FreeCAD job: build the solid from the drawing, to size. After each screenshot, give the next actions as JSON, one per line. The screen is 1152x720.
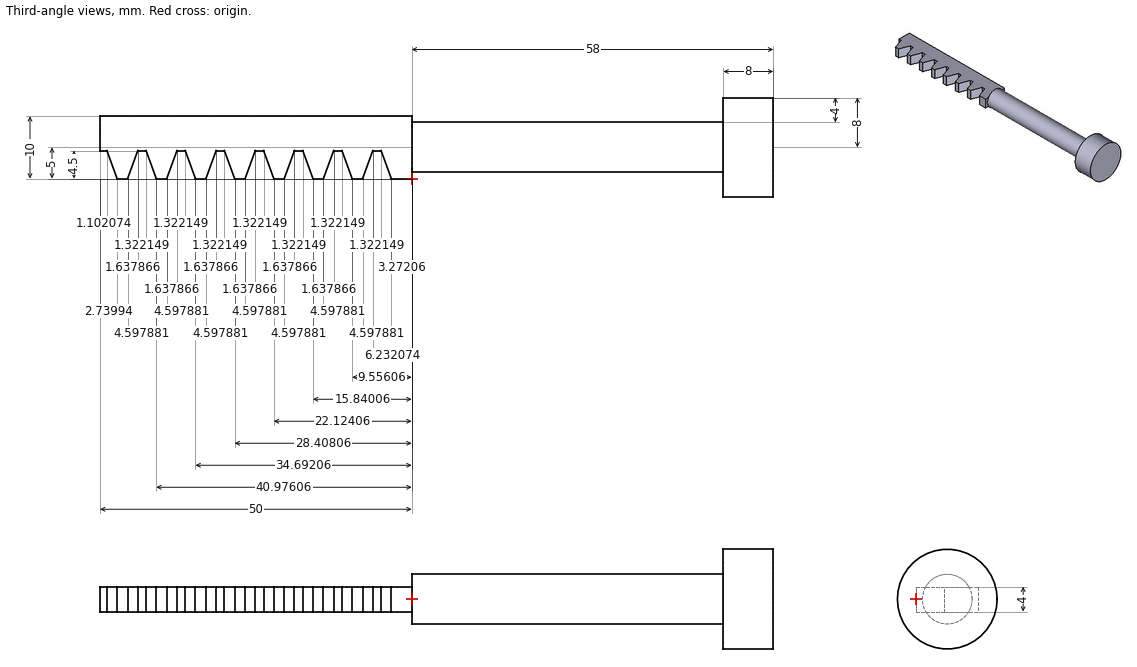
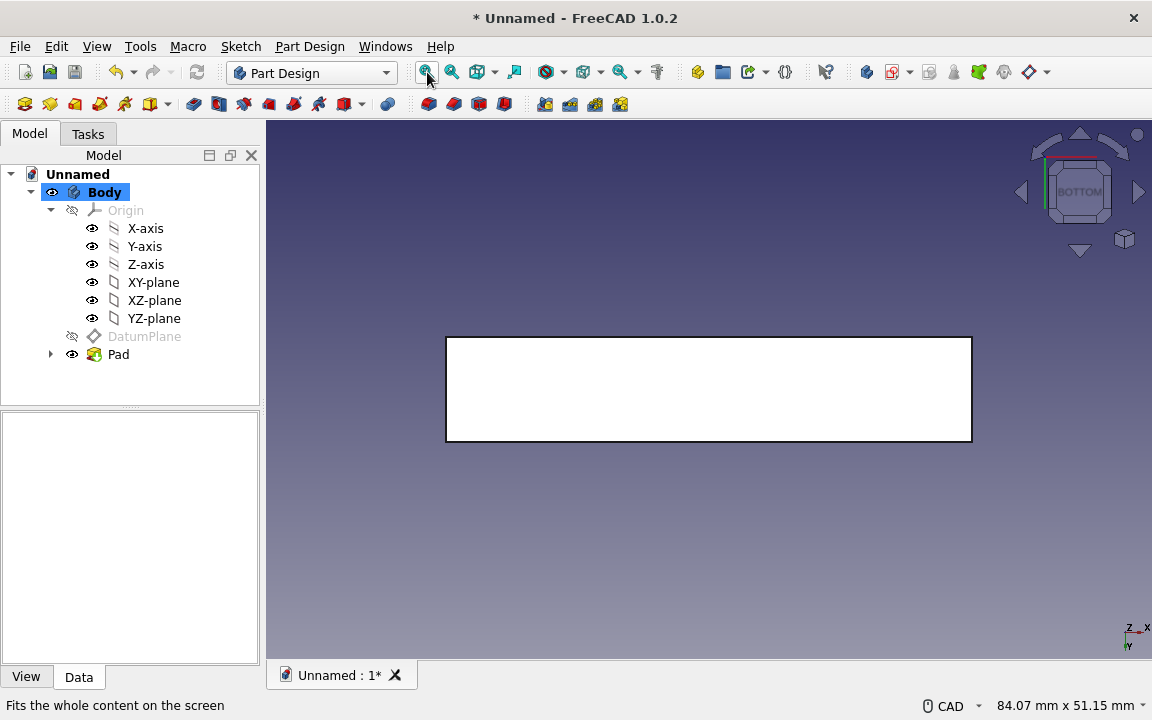
{"action": "left_click", "coordinate": [860, 388]}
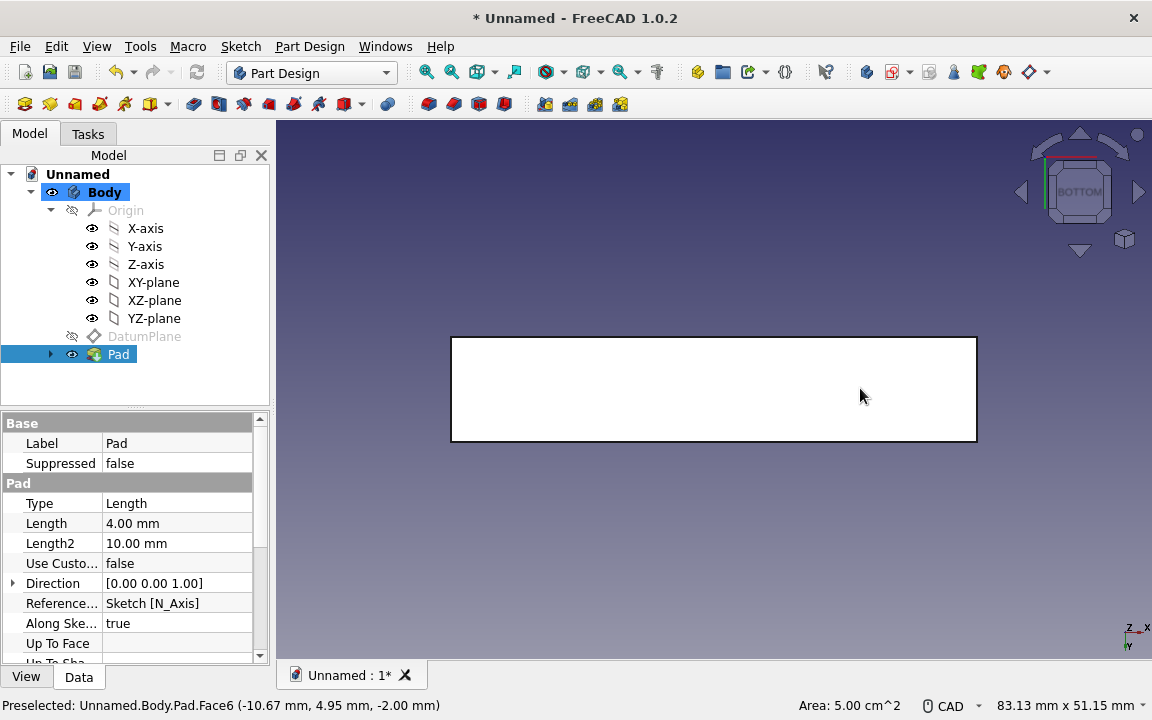
{"action": "left_click", "coordinate": [892, 72]}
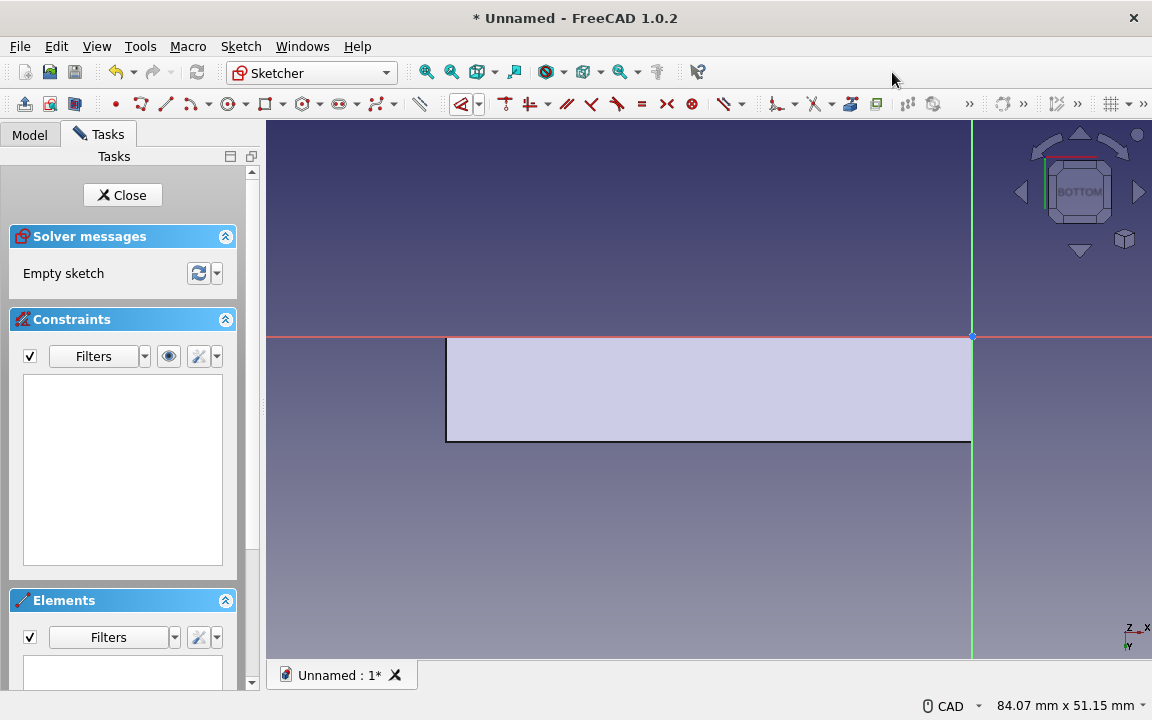
{"action": "scroll", "coordinate": [497, 356], "scroll_direction": "up", "scroll_amount": 10}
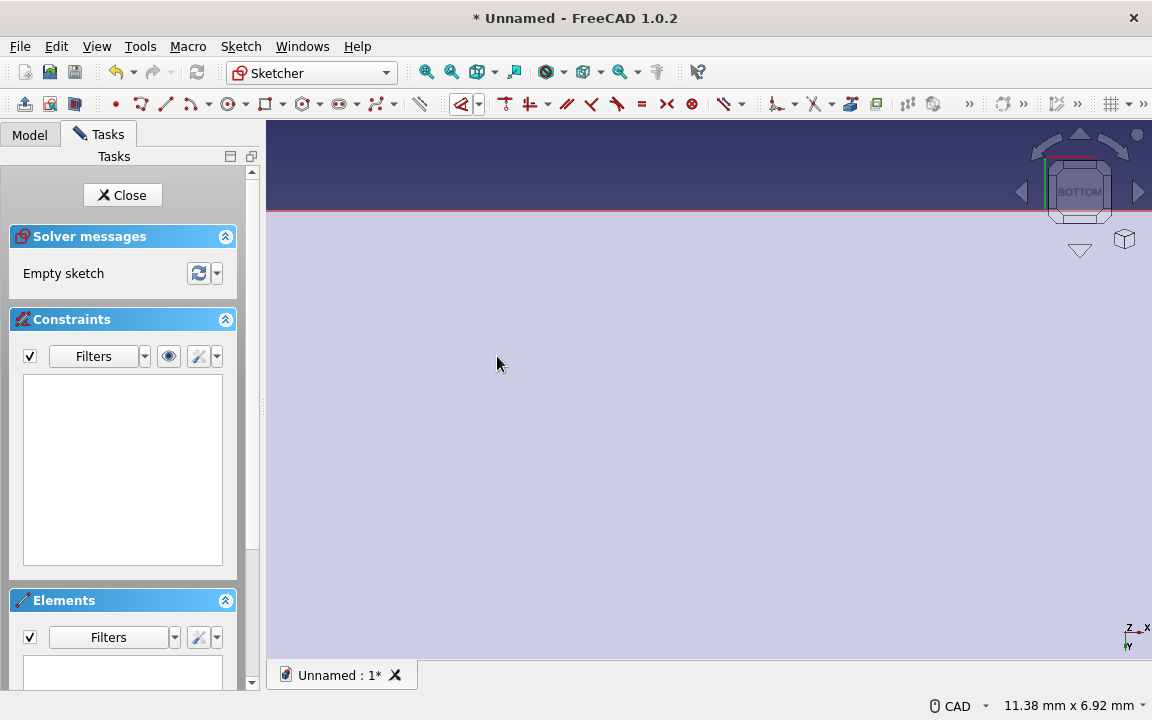
{"action": "left_click", "coordinate": [141, 104]}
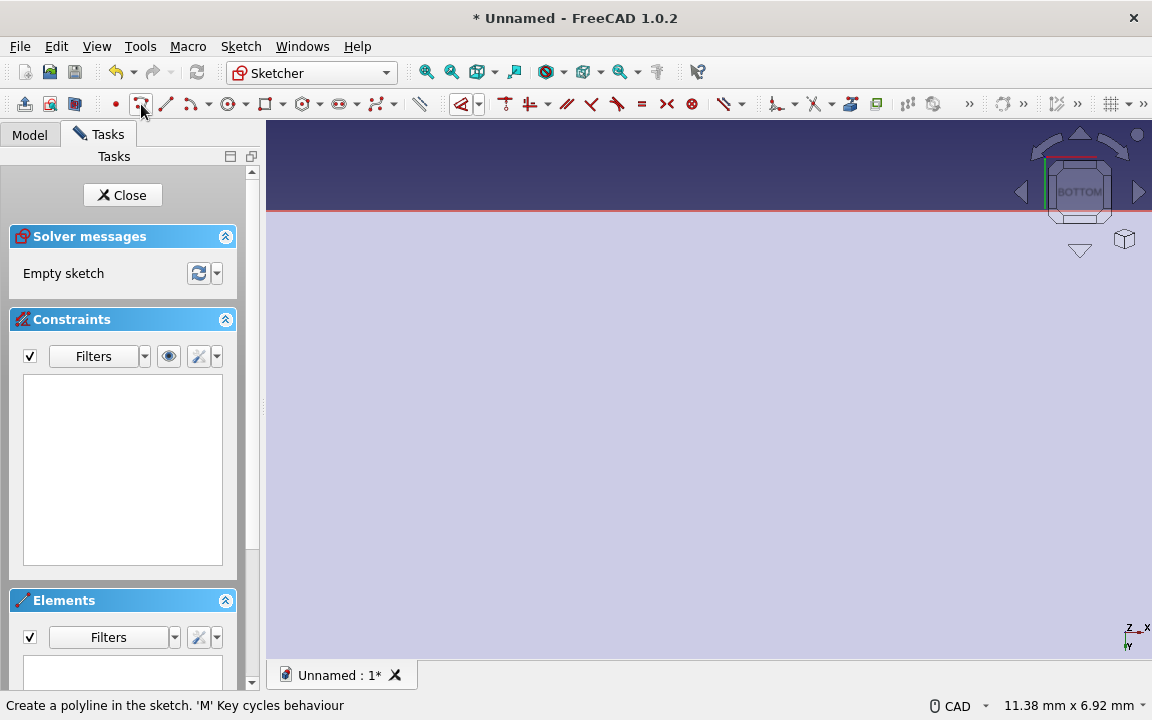
{"action": "left_click", "coordinate": [818, 211]}
{"action": "left_click", "coordinate": [460, 220]}
{"action": "left_click", "coordinate": [587, 562]}
{"action": "left_click", "coordinate": [690, 562]}
{"action": "left_click", "coordinate": [818, 211]}
{"action": "key", "text": "Escape"}
{"action": "key", "text": "Escape"}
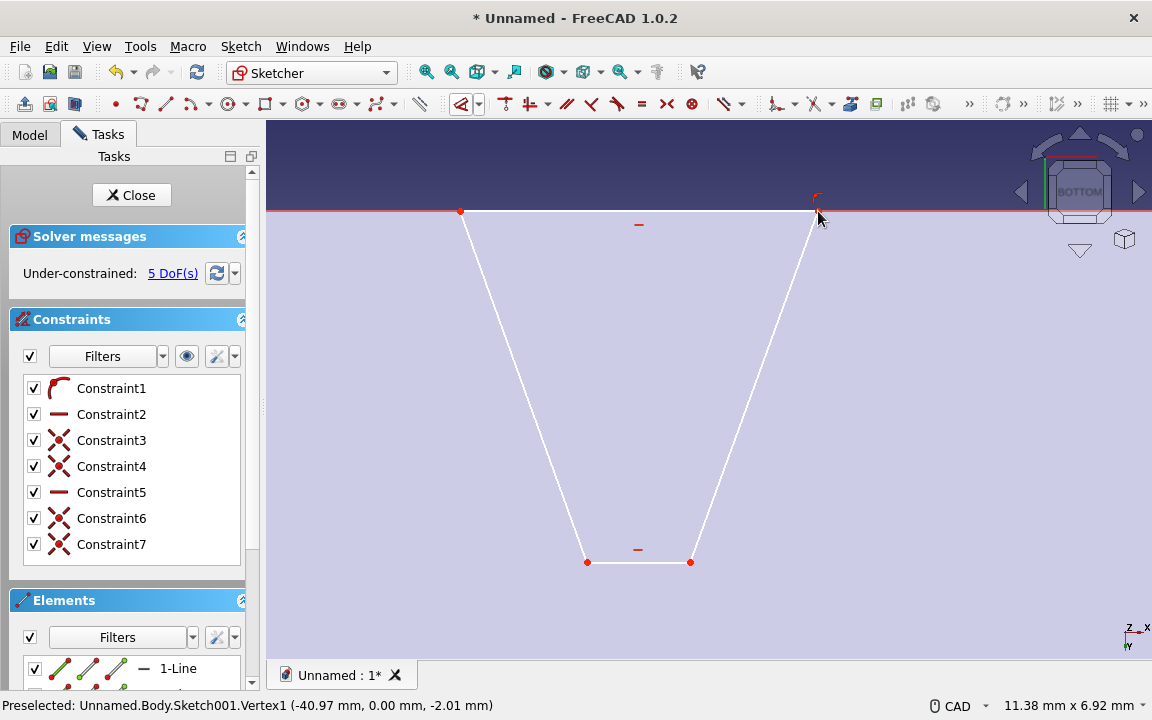
{"action": "left_click", "coordinate": [460, 104]}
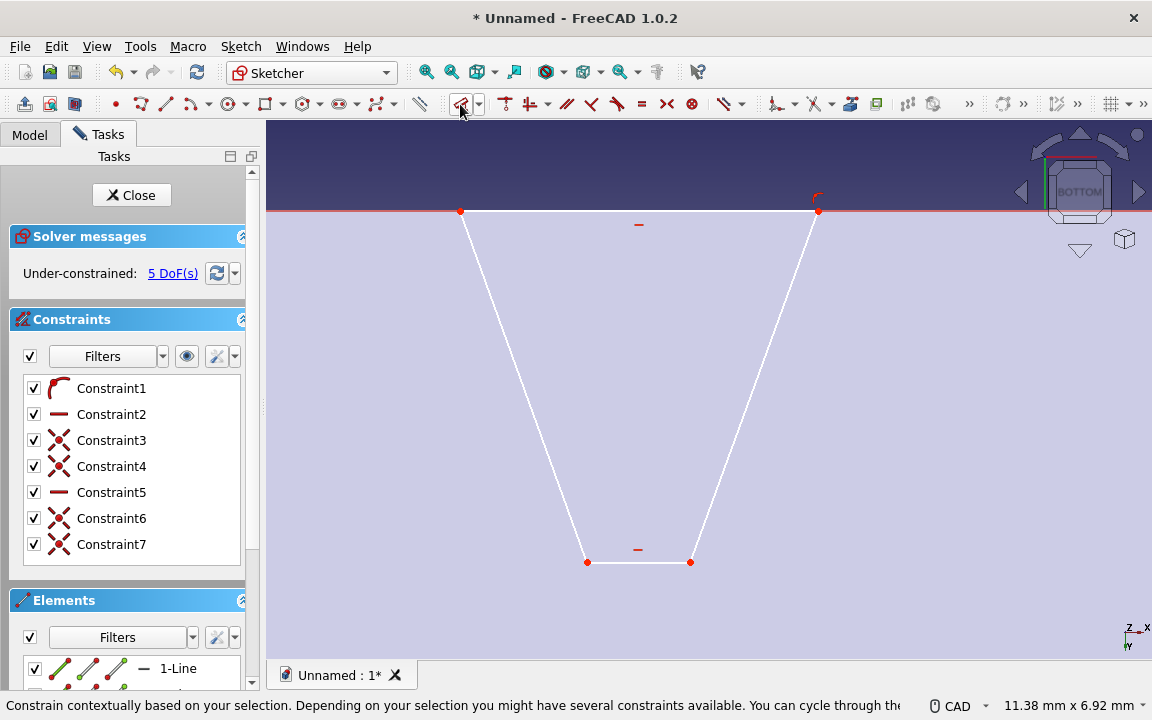
{"action": "left_click", "coordinate": [587, 563]}
{"action": "left_click", "coordinate": [553, 387]}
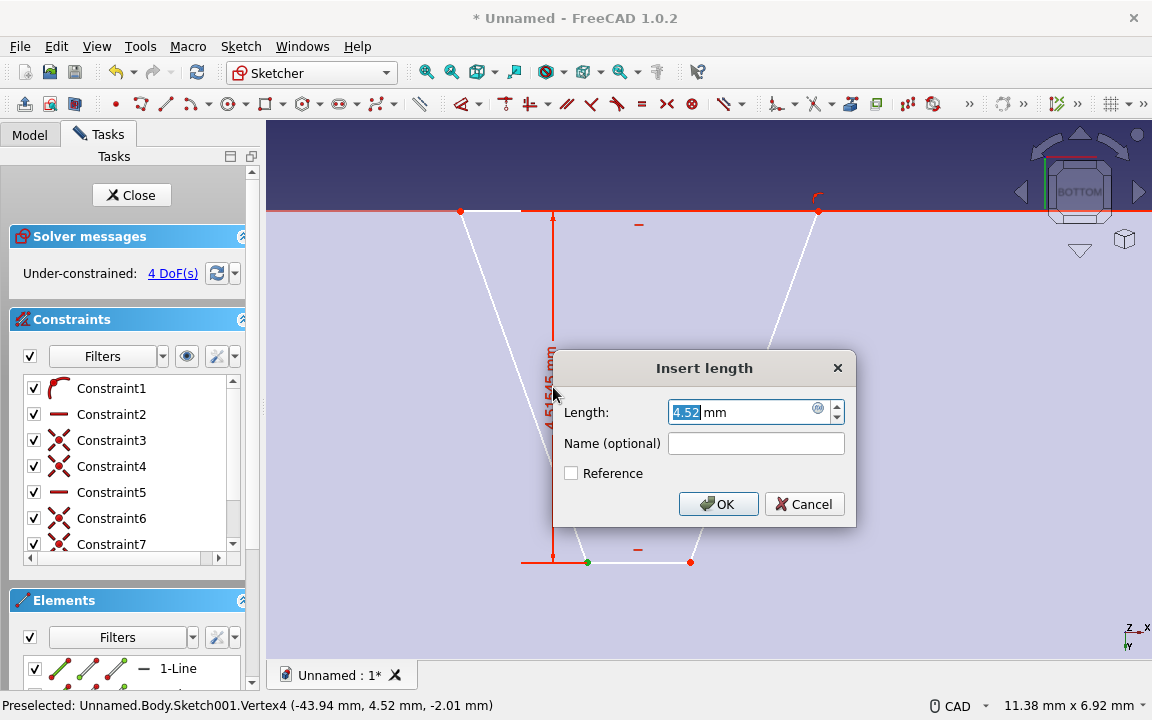
{"action": "type", "text": "4.5"}
{"action": "key", "text": "Return"}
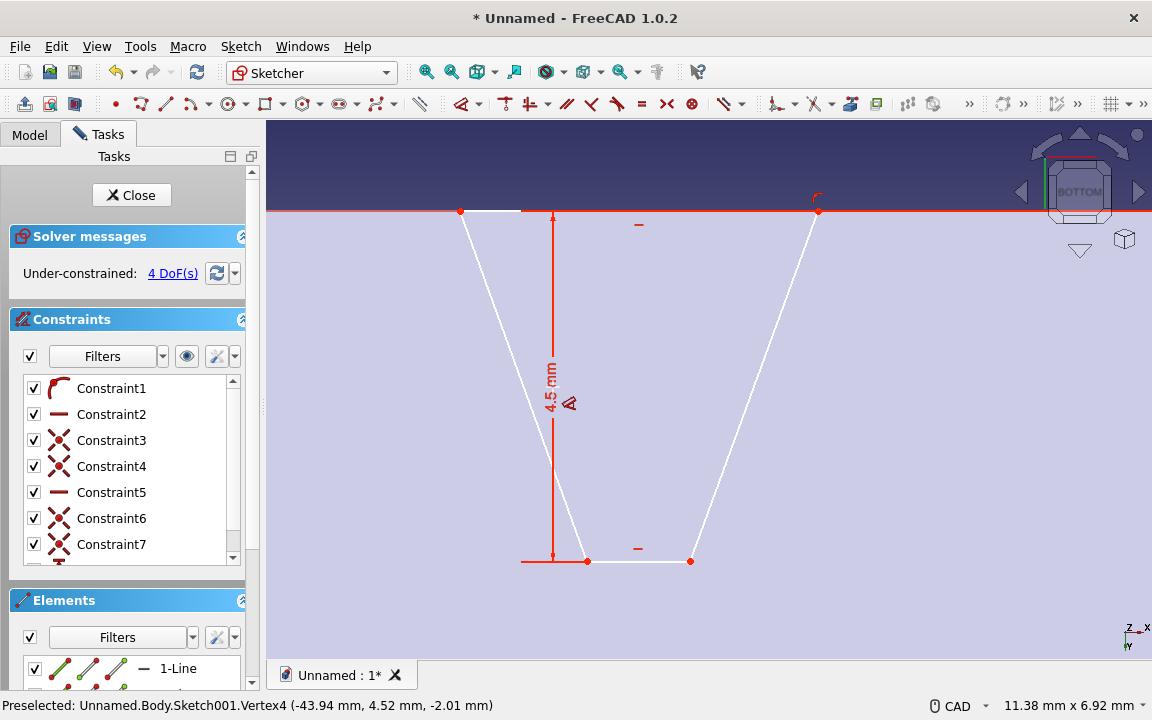
{"action": "left_click", "coordinate": [711, 211]}
{"action": "left_click", "coordinate": [639, 177]}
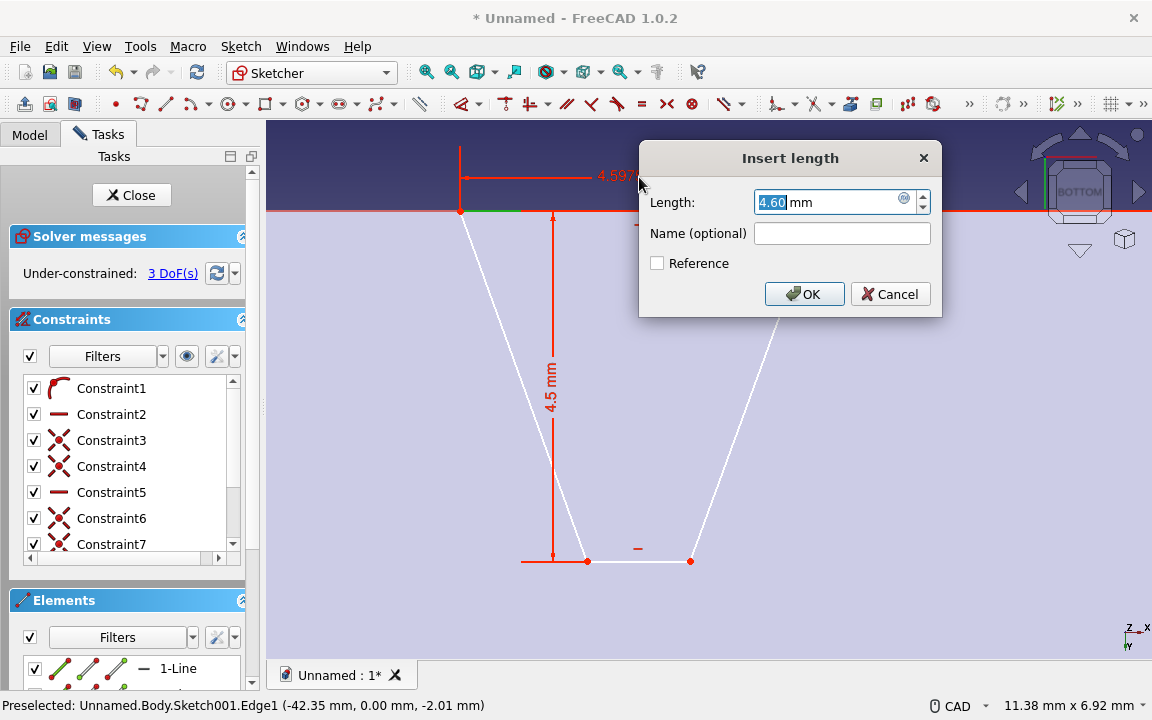
{"action": "type", "text": "4.597881"}
{"action": "key", "text": "Return"}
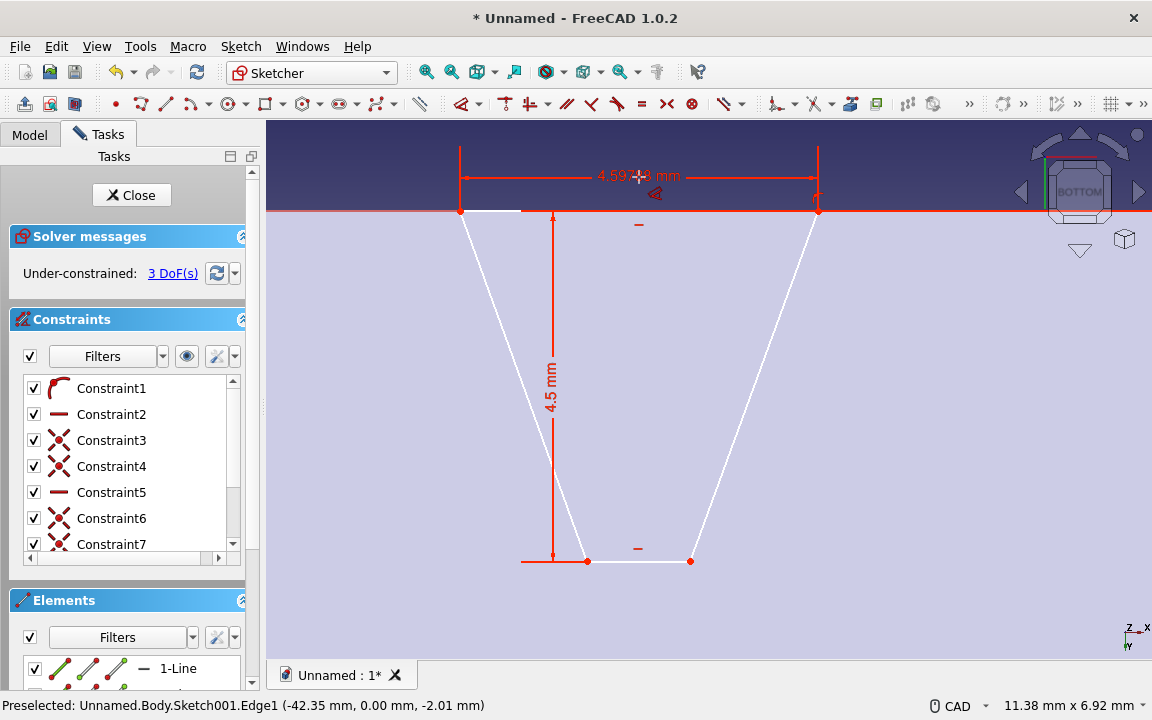
{"action": "left_click", "coordinate": [618, 562]}
{"action": "left_click", "coordinate": [639, 596]}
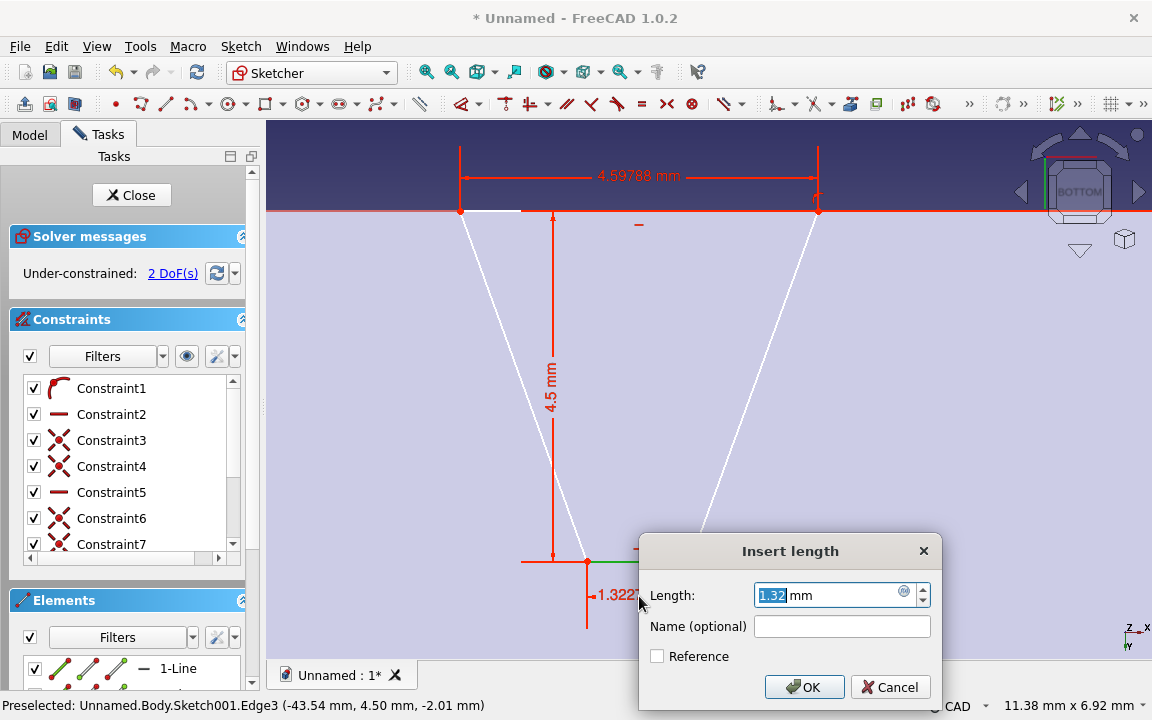
{"action": "type", "text": "1.322149"}
{"action": "key", "text": "Return"}